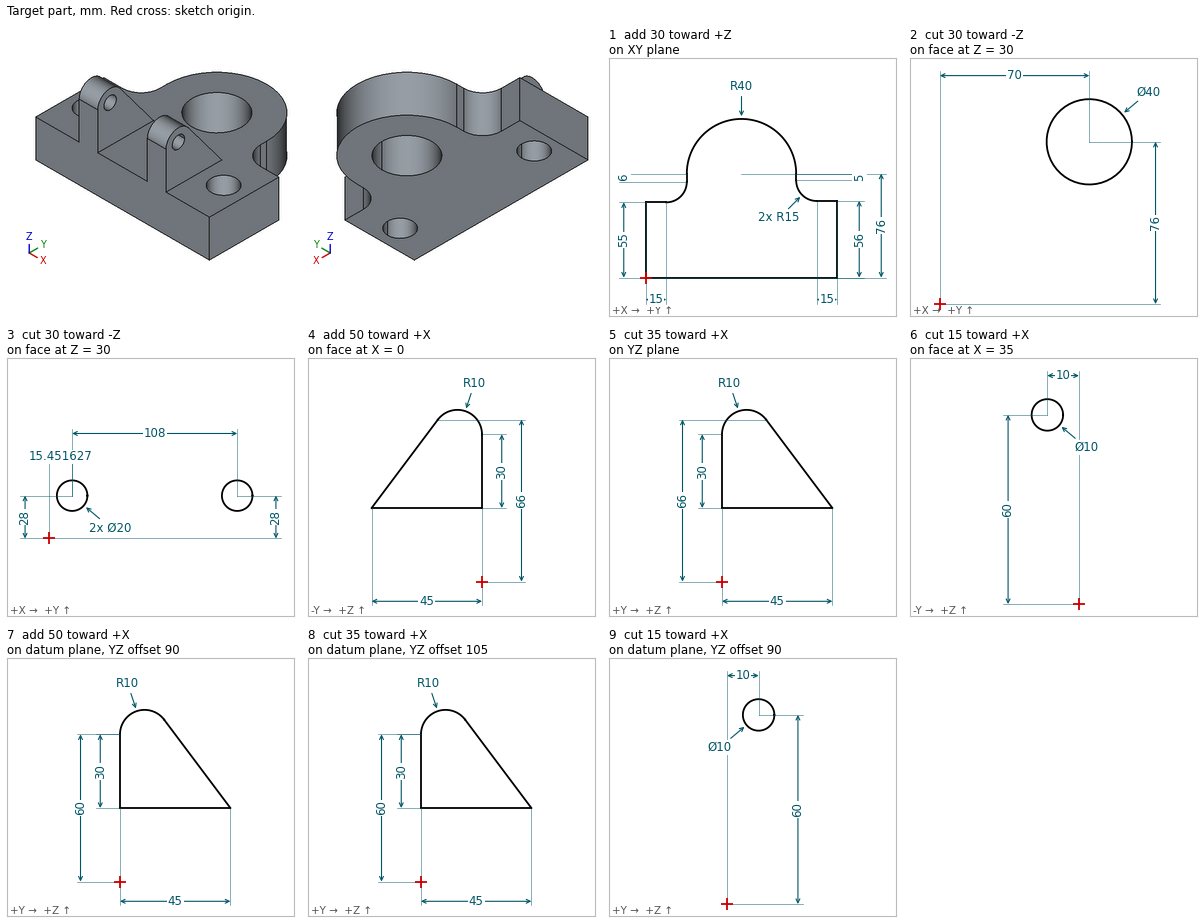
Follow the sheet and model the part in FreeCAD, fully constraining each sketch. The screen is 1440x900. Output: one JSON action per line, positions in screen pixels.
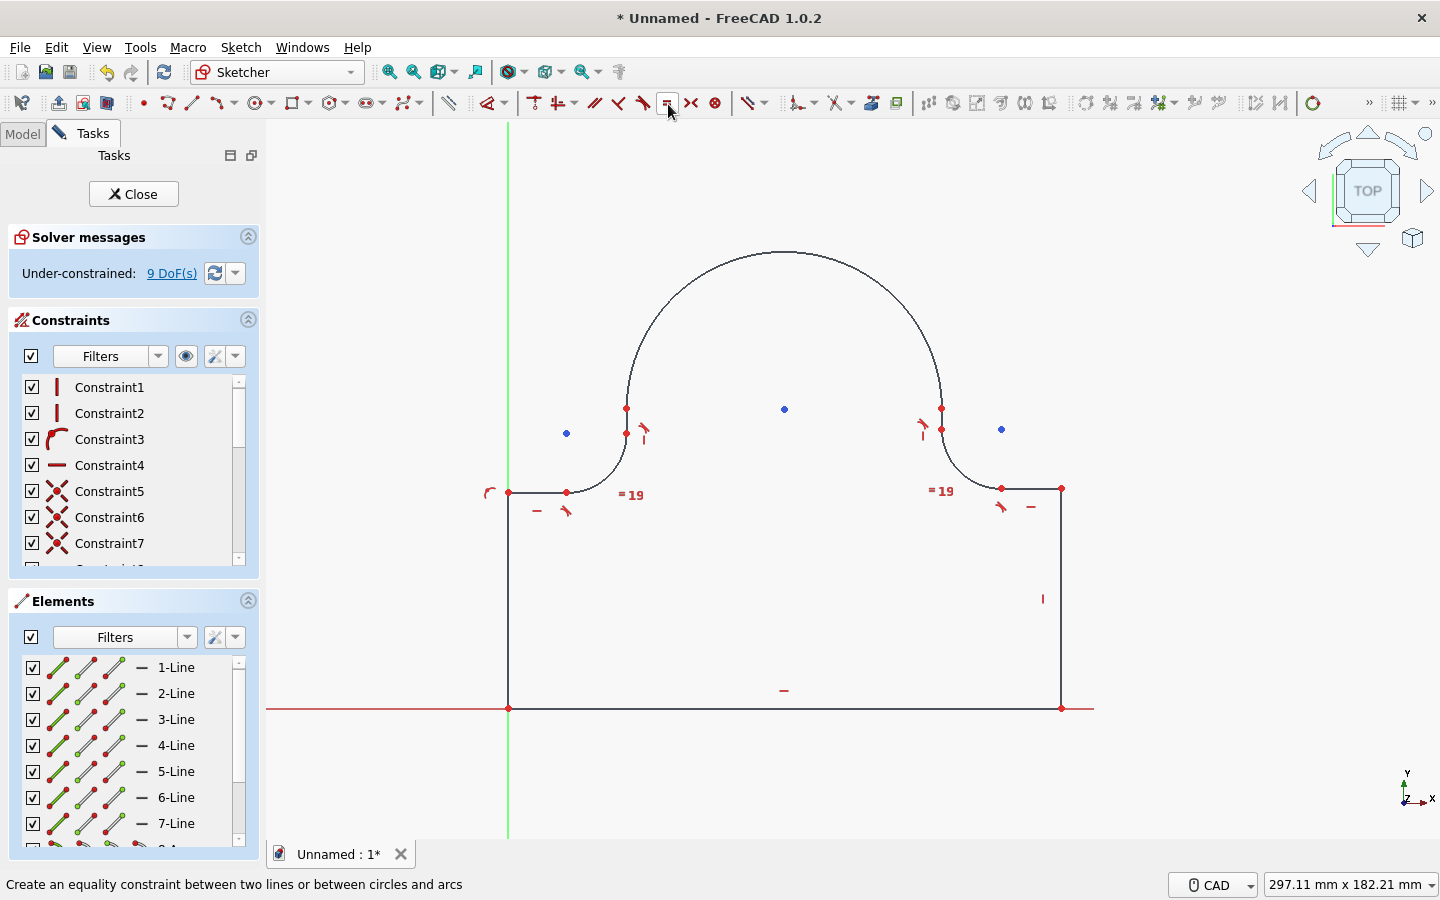
{"action": "left_click", "coordinate": [877, 282]}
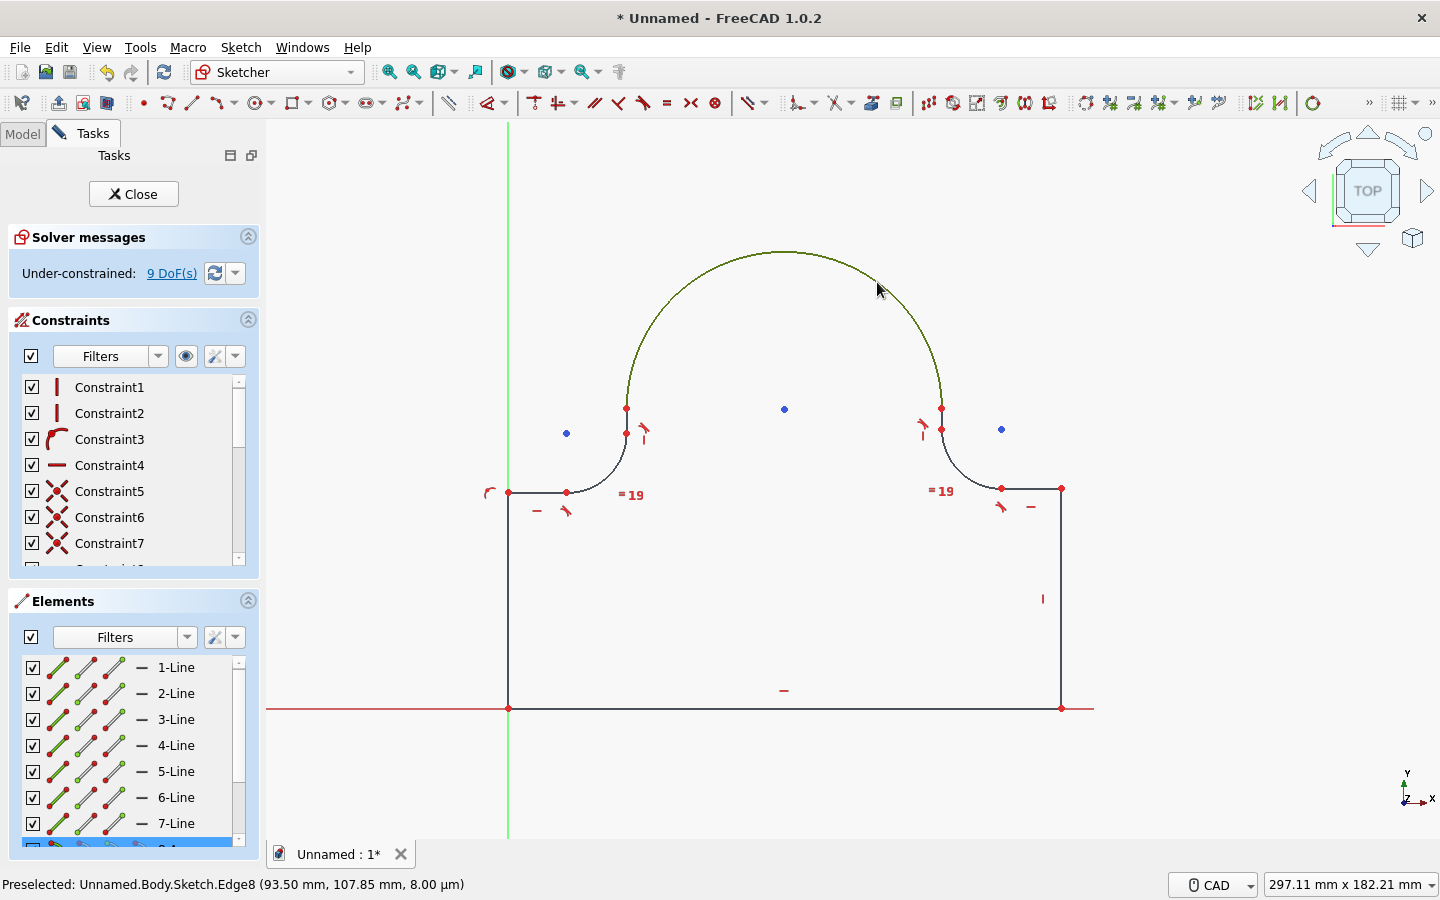
{"action": "key", "text": "k r"}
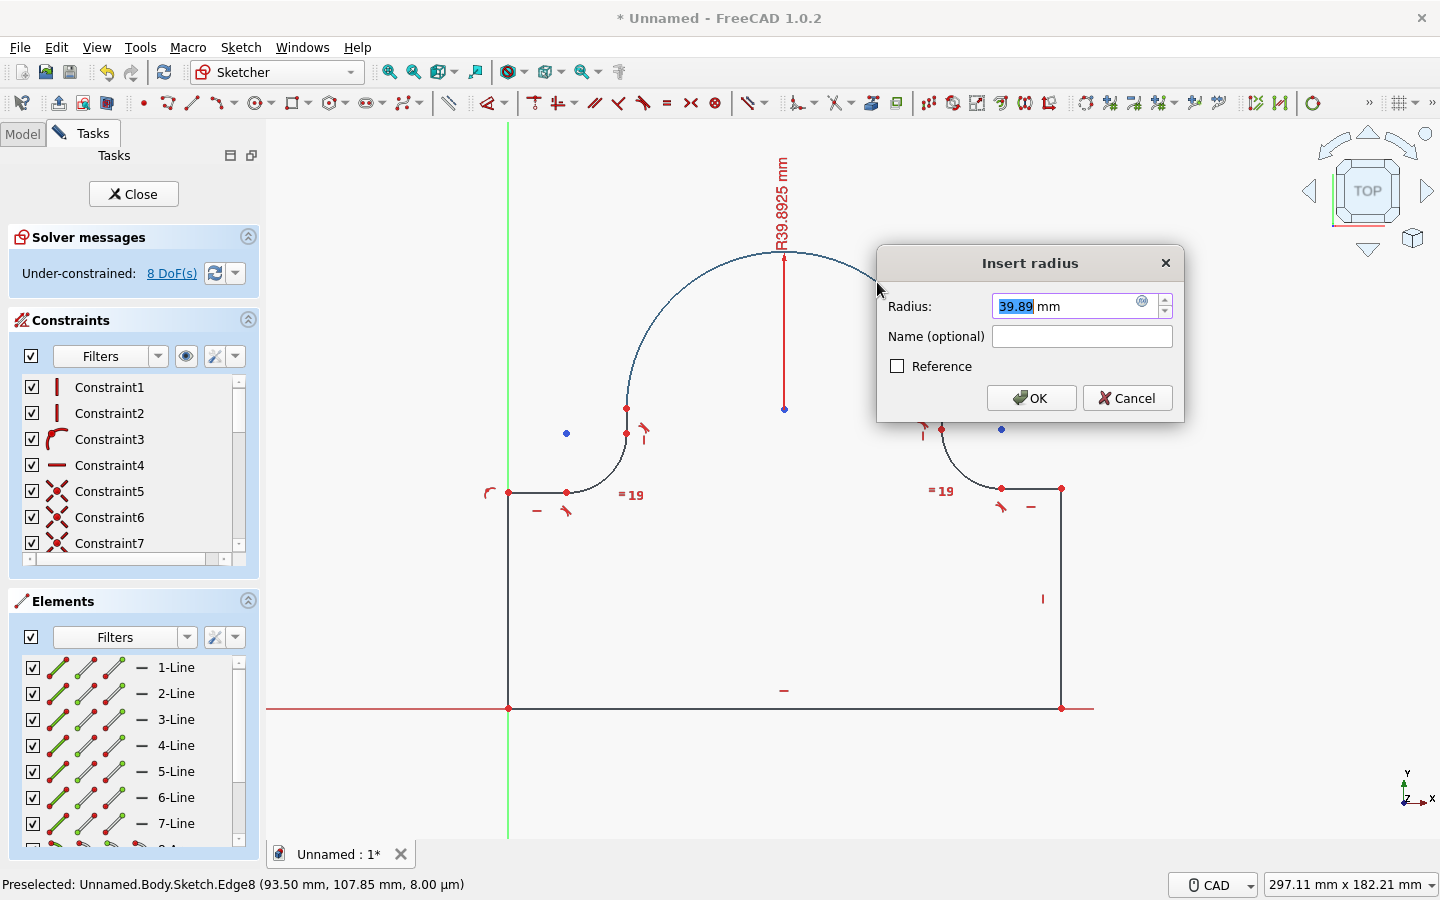
{"action": "type", "text": "40"}
{"action": "key", "text": "Return"}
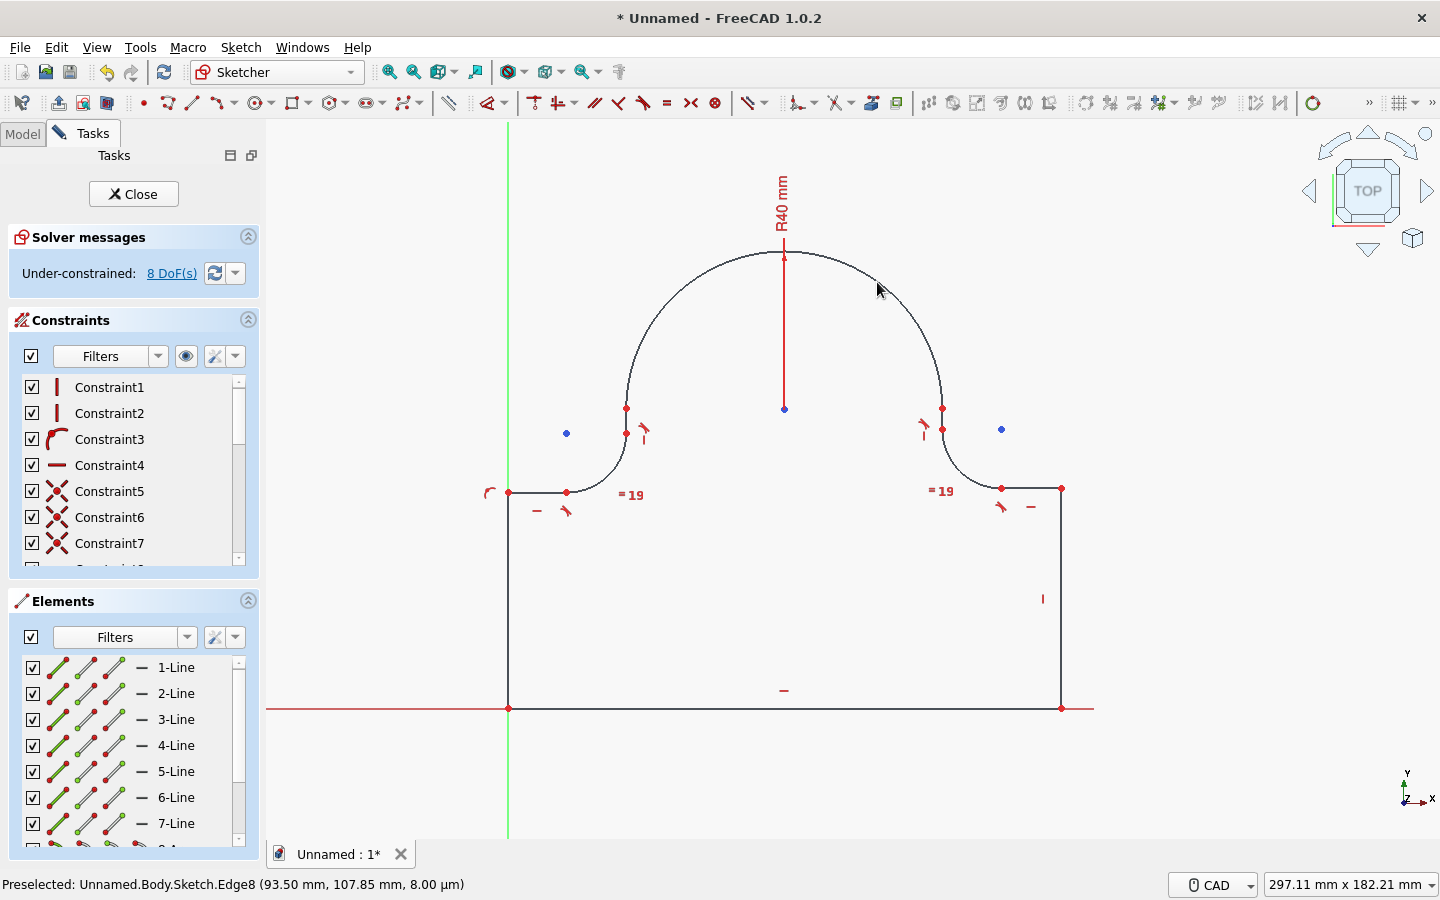
{"action": "left_click", "coordinate": [594, 486]}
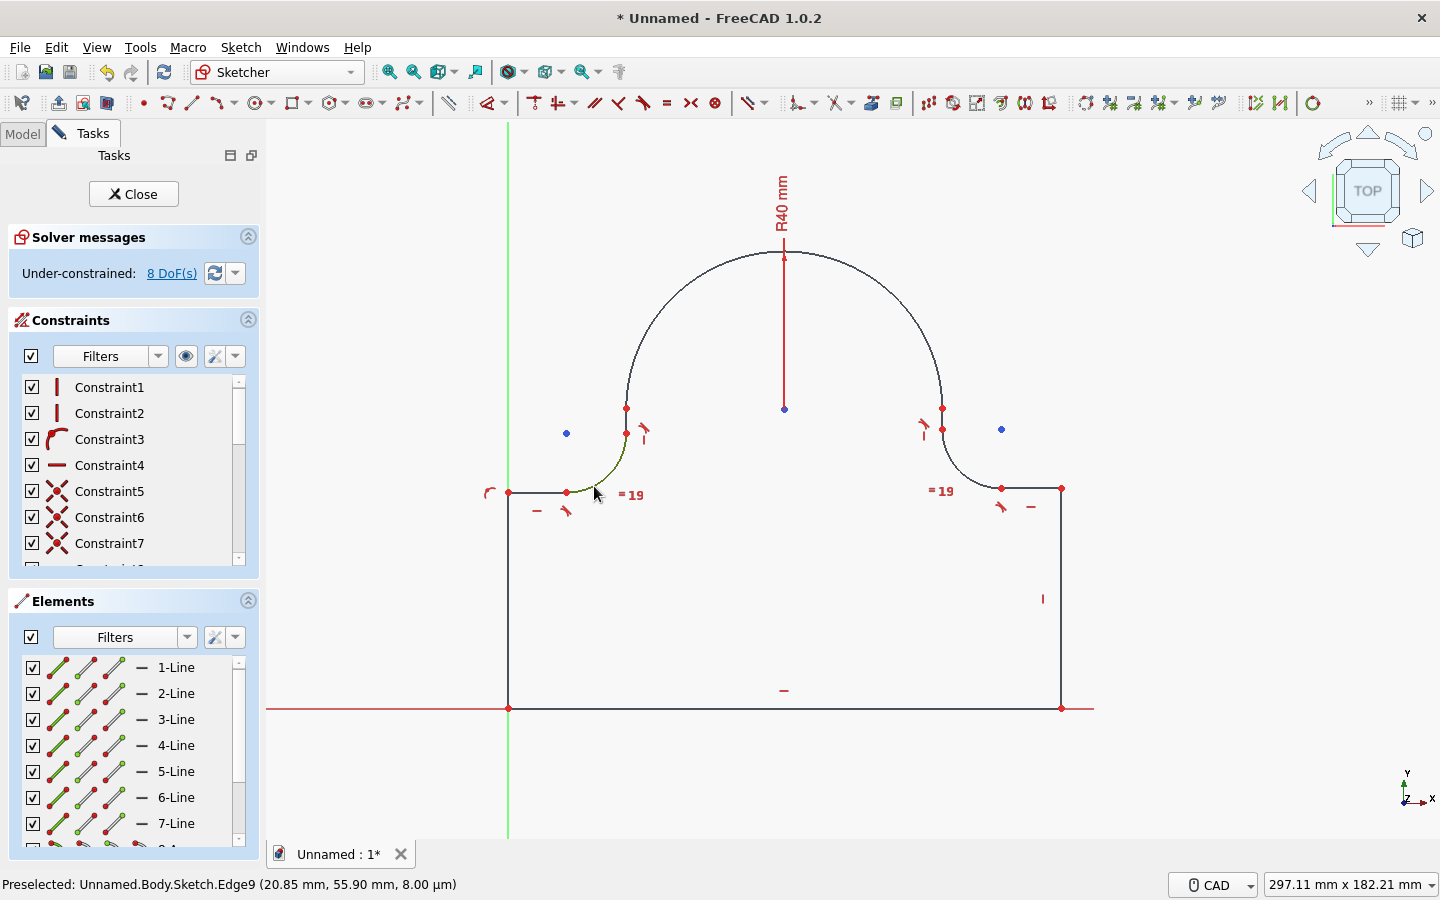
{"action": "key", "text": "k r"}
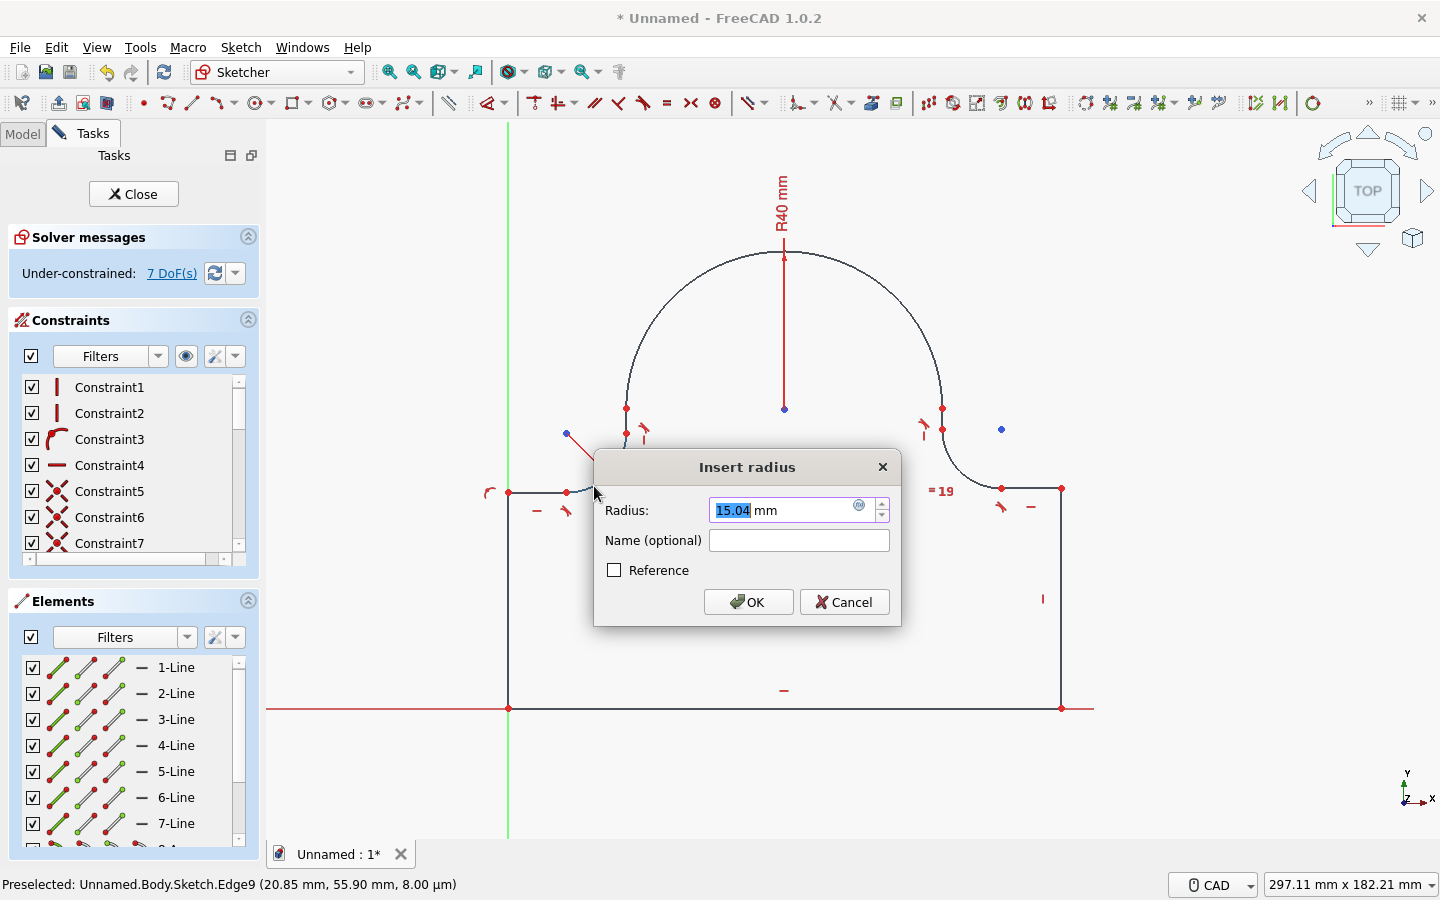
{"action": "type", "text": "15"}
{"action": "key", "text": "Return"}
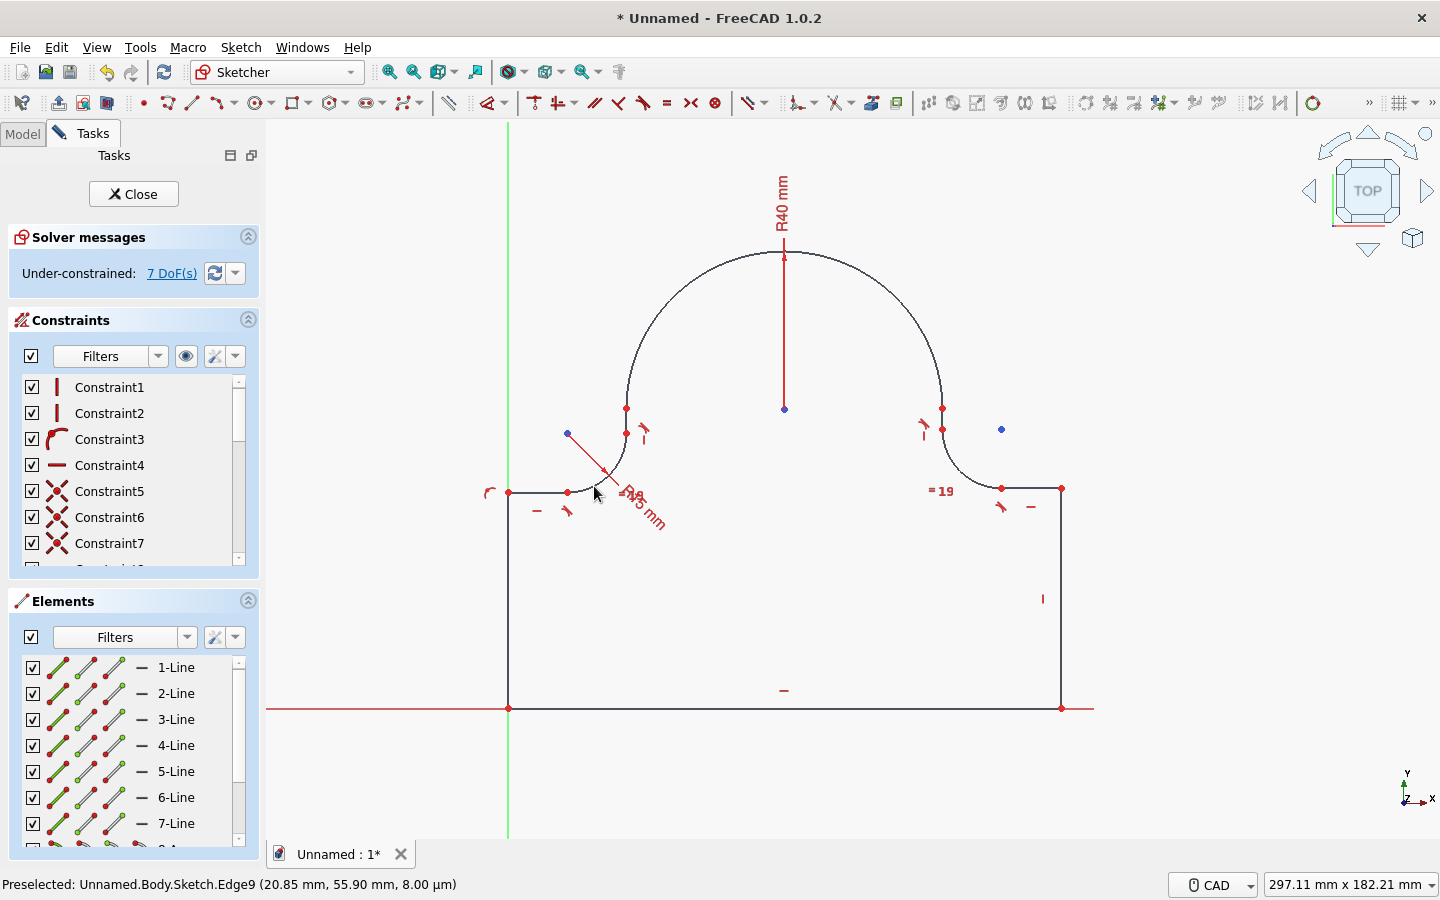
{"action": "scroll", "coordinate": [942, 419], "scroll_direction": "up", "scroll_amount": 4}